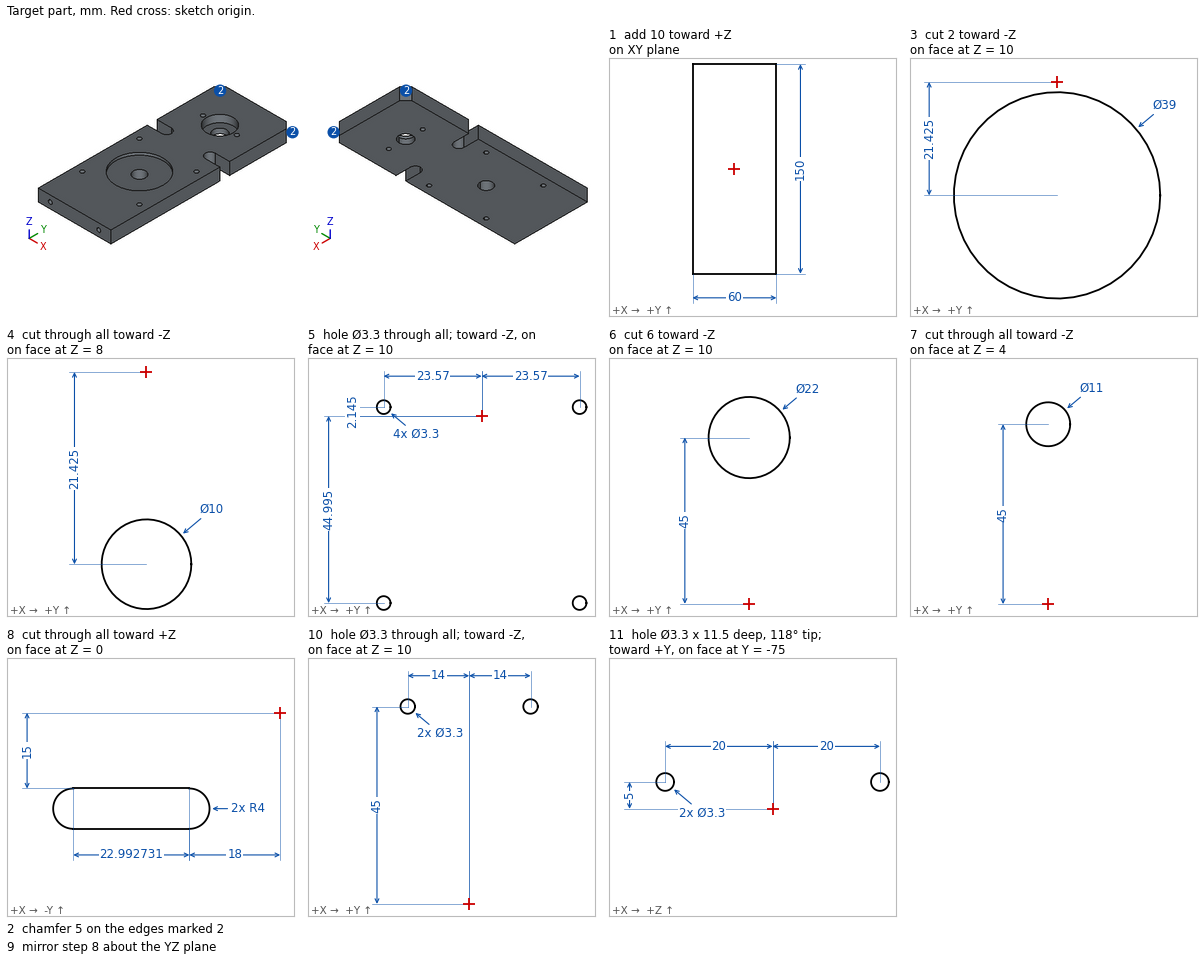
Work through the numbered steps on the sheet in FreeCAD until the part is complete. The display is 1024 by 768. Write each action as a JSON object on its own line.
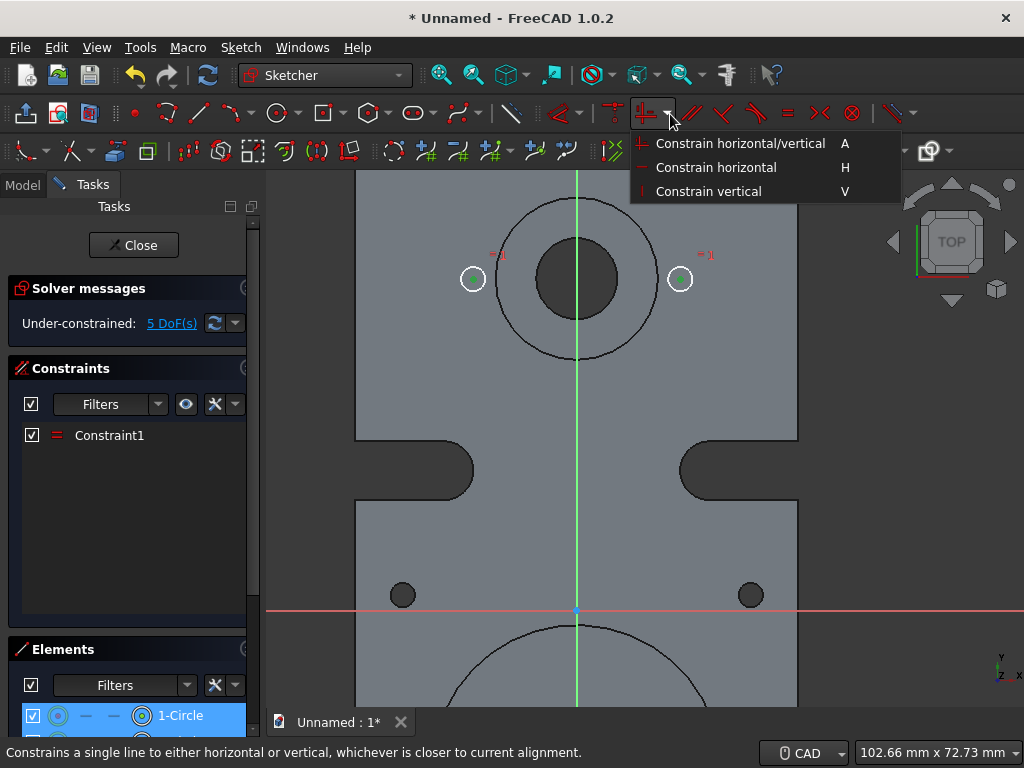
{"action": "left_click", "coordinate": [766, 167]}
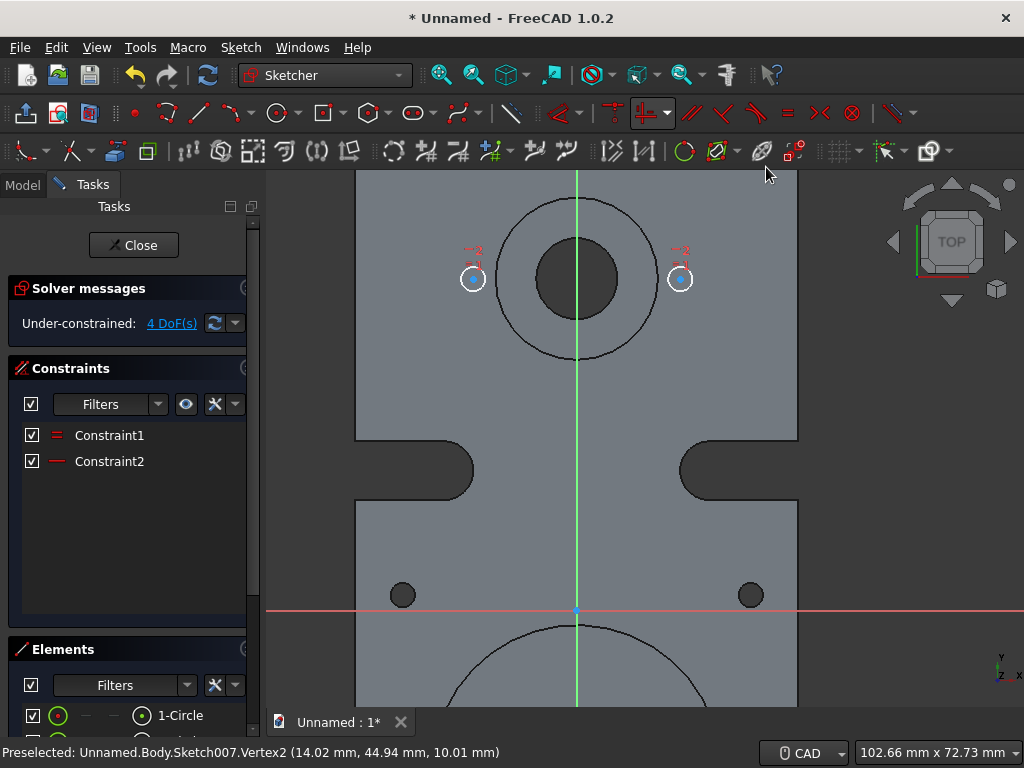
{"action": "left_click", "coordinate": [558, 114]}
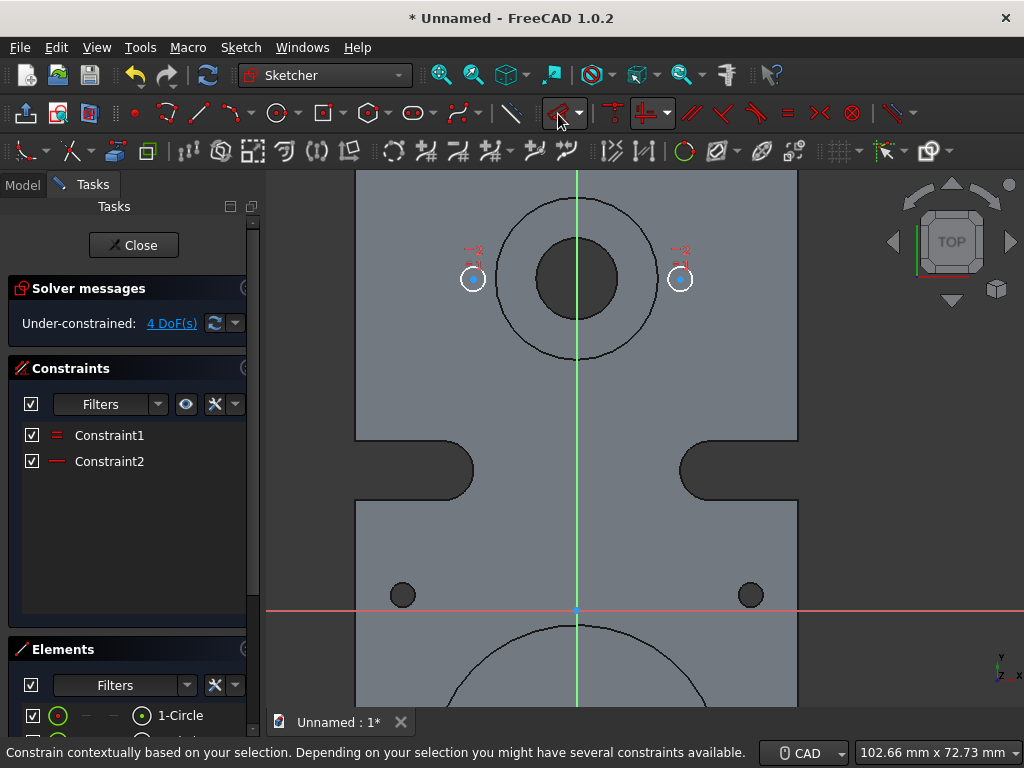
{"action": "scroll", "coordinate": [482, 271], "scroll_direction": "up", "scroll_amount": 3}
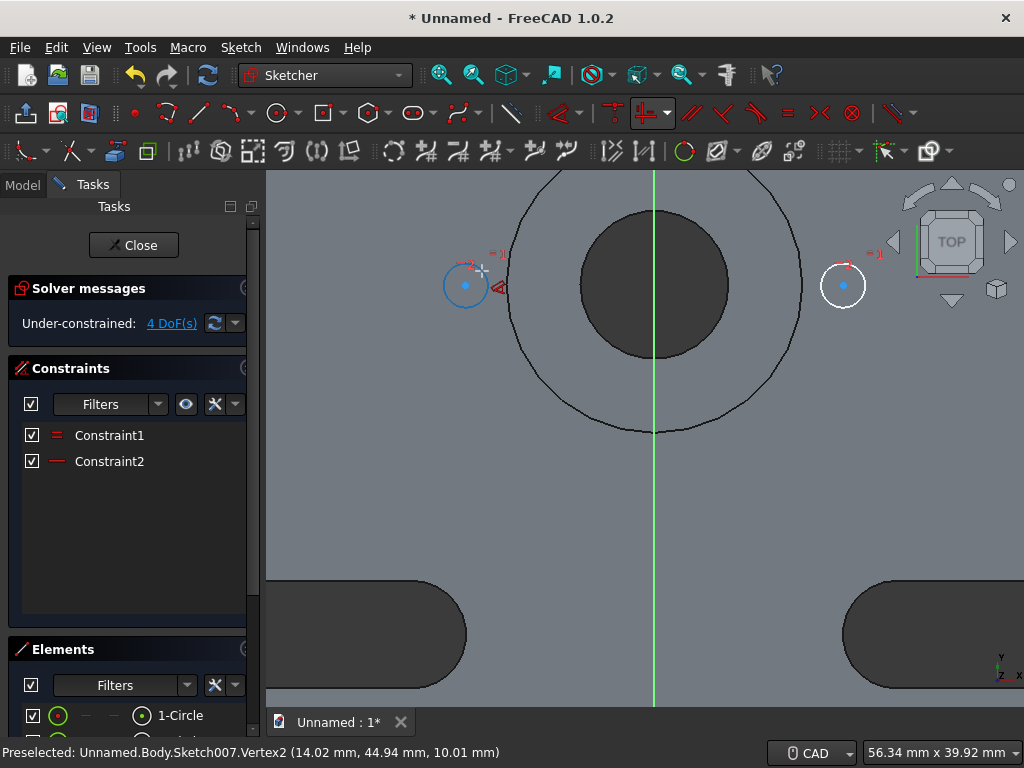
{"action": "left_click", "coordinate": [481, 270]}
{"action": "left_click", "coordinate": [503, 247]}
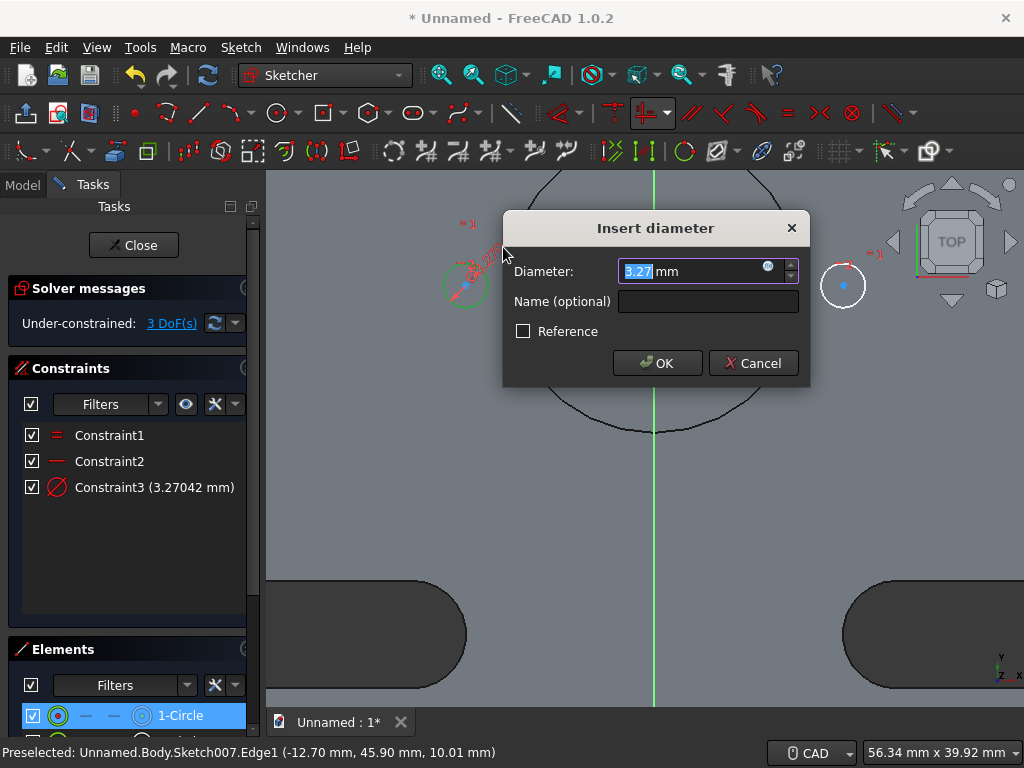
{"action": "type", "text": "3.3"}
{"action": "key", "text": "Return"}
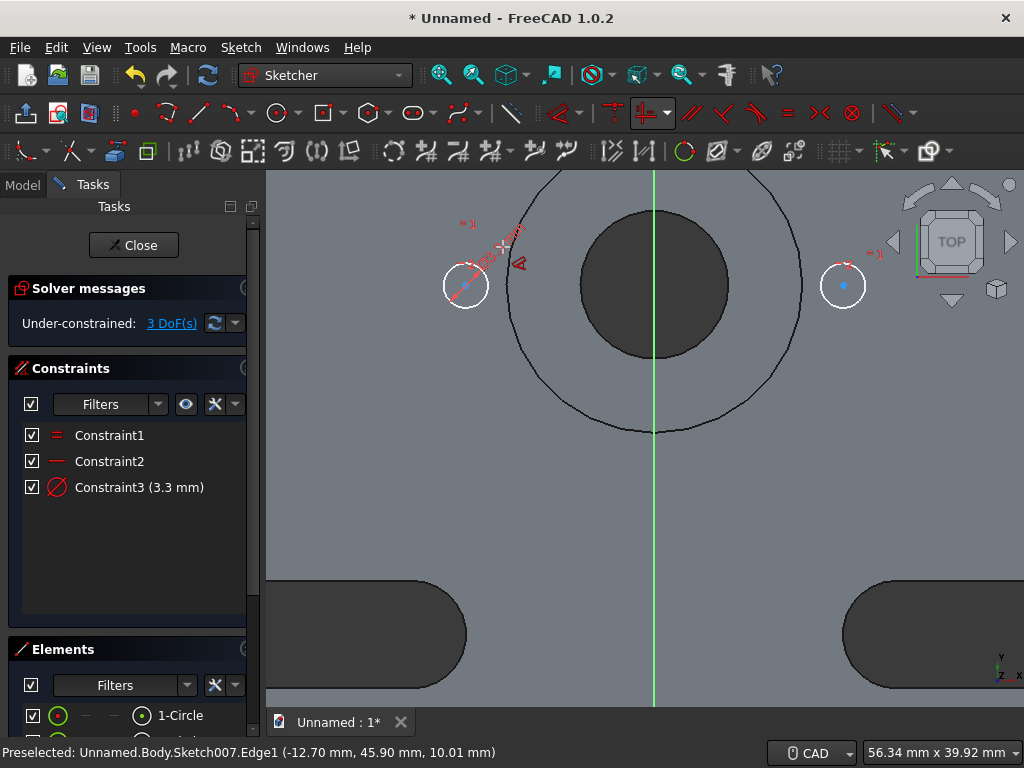
{"action": "left_click", "coordinate": [466, 286]}
{"action": "left_click", "coordinate": [604, 252]}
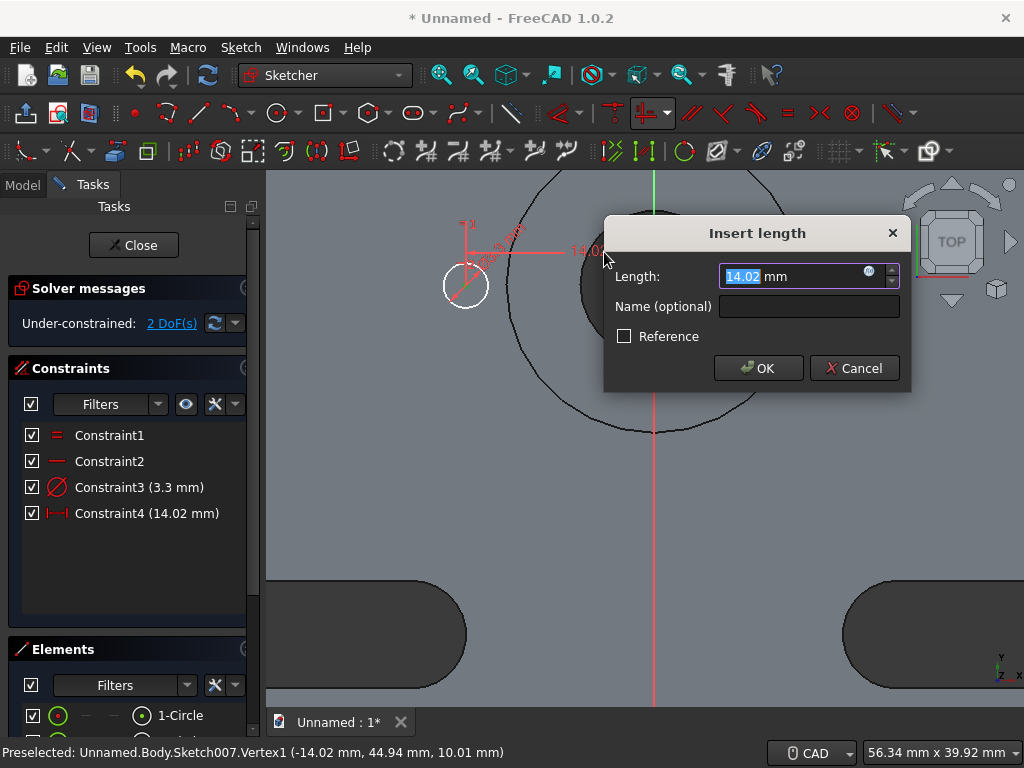
{"action": "type", "text": "14"}
{"action": "key", "text": "Return"}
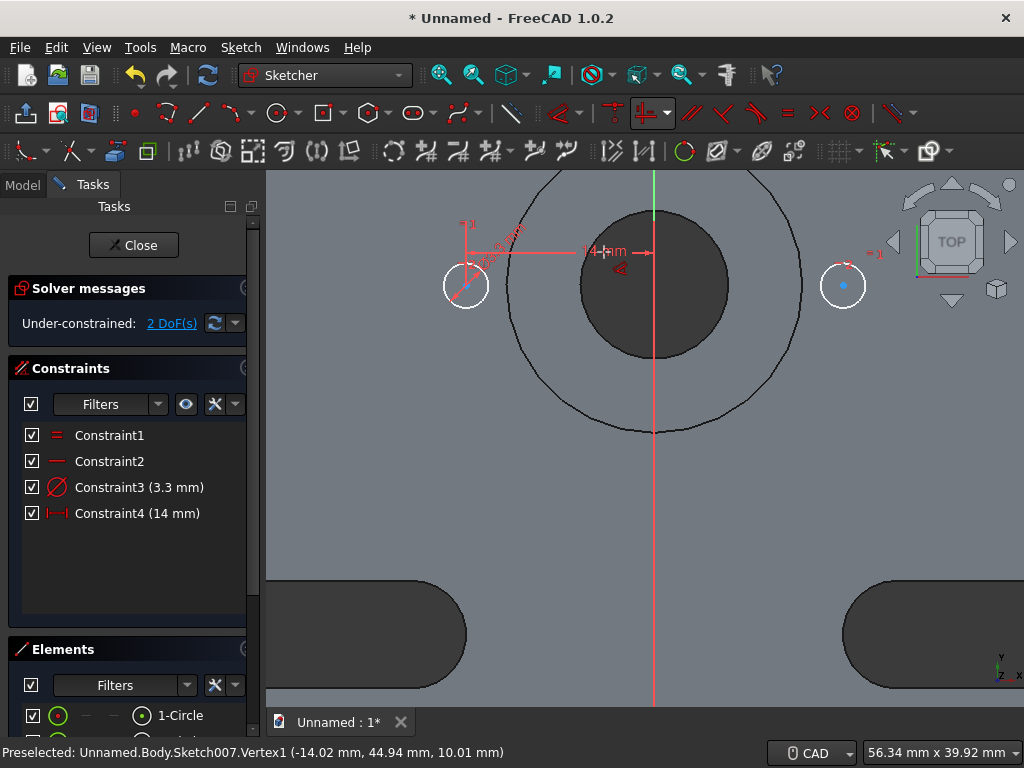
{"action": "left_click", "coordinate": [466, 286]}
{"action": "left_click", "coordinate": [432, 482]}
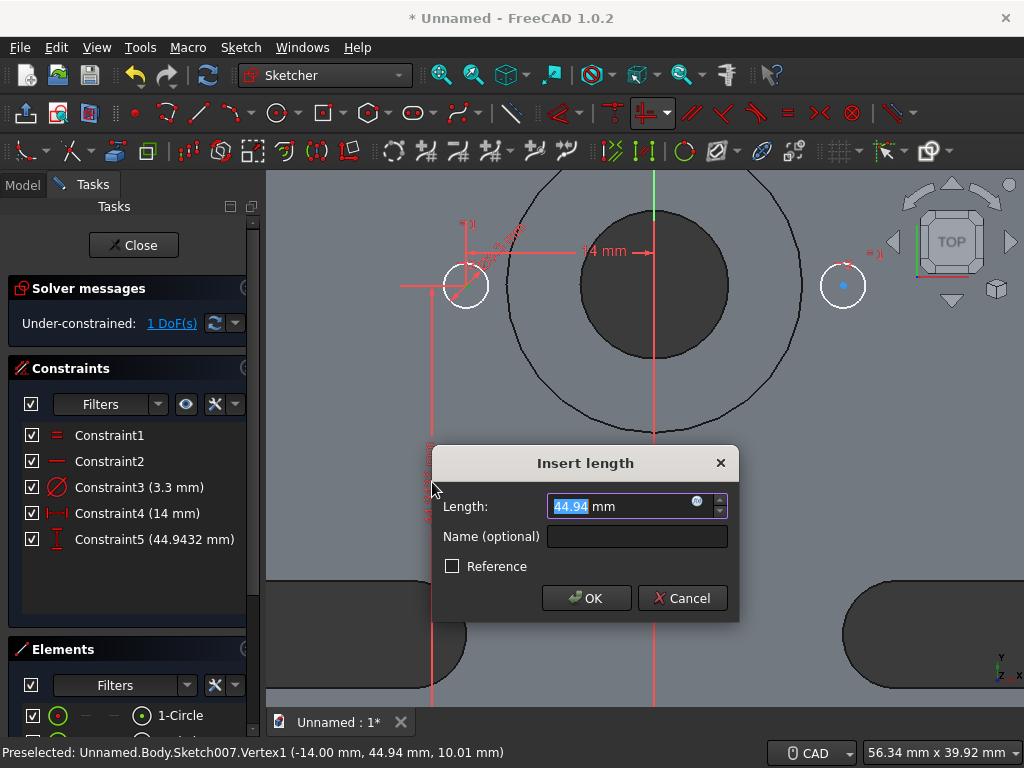
{"action": "type", "text": "45"}
{"action": "key", "text": "Return"}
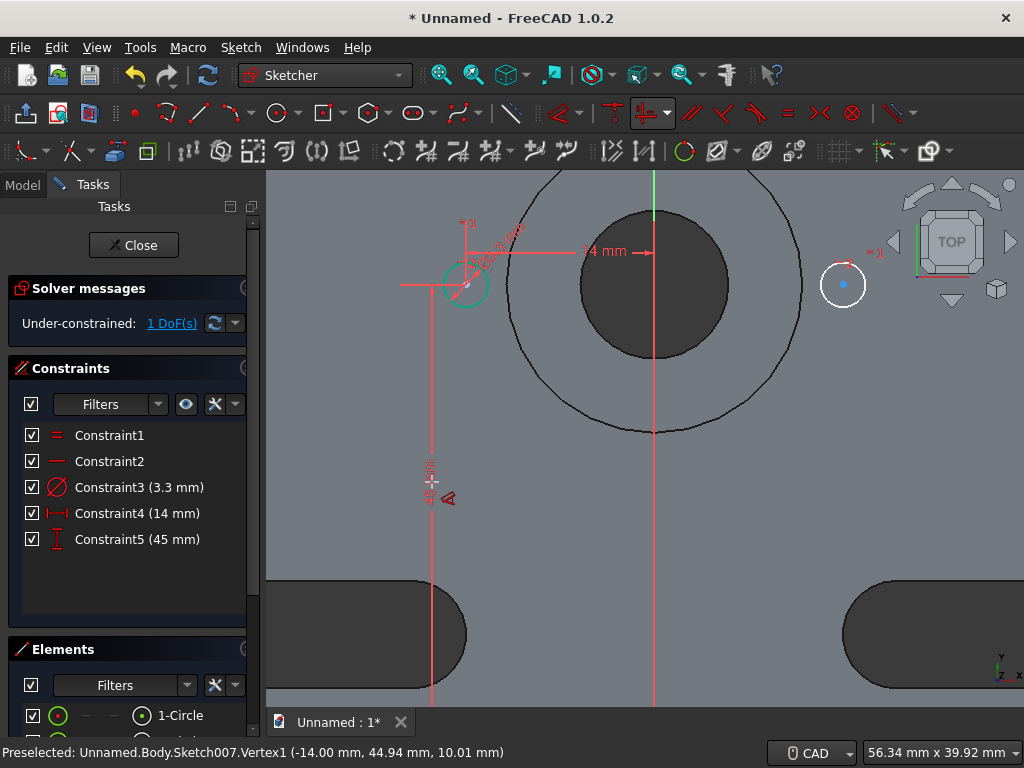
{"action": "left_click", "coordinate": [843, 285]}
{"action": "left_click", "coordinate": [749, 251]}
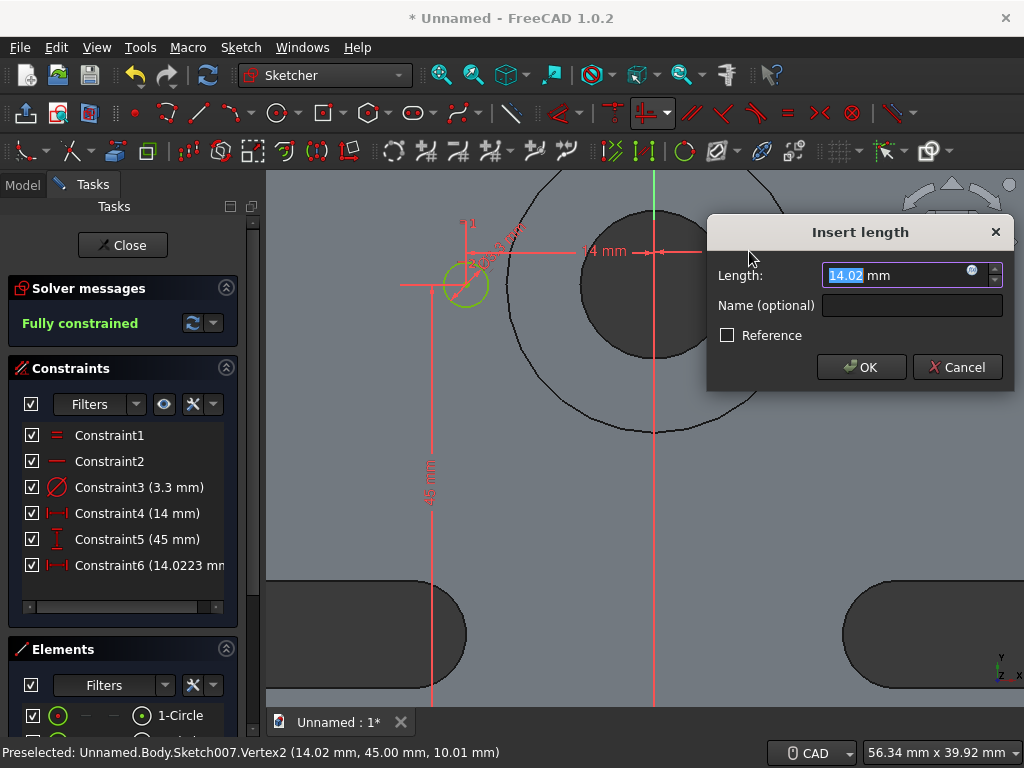
{"action": "type", "text": "14"}
{"action": "key", "text": "Return"}
{"action": "key", "text": "Escape"}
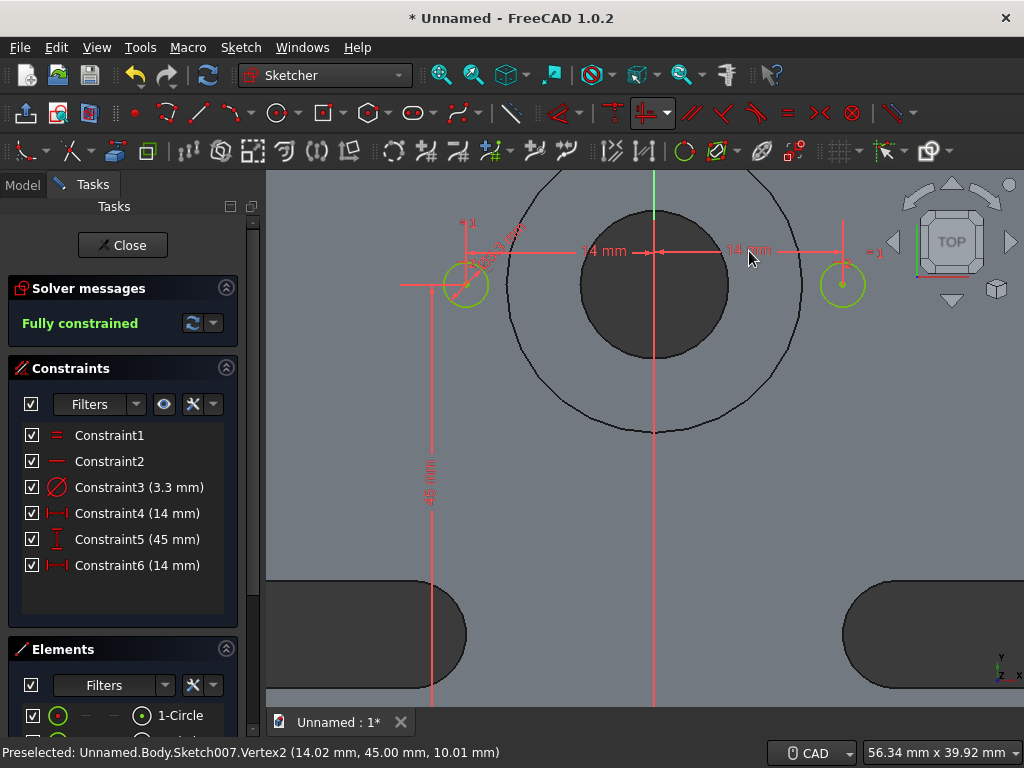
{"action": "left_click", "coordinate": [123, 245]}